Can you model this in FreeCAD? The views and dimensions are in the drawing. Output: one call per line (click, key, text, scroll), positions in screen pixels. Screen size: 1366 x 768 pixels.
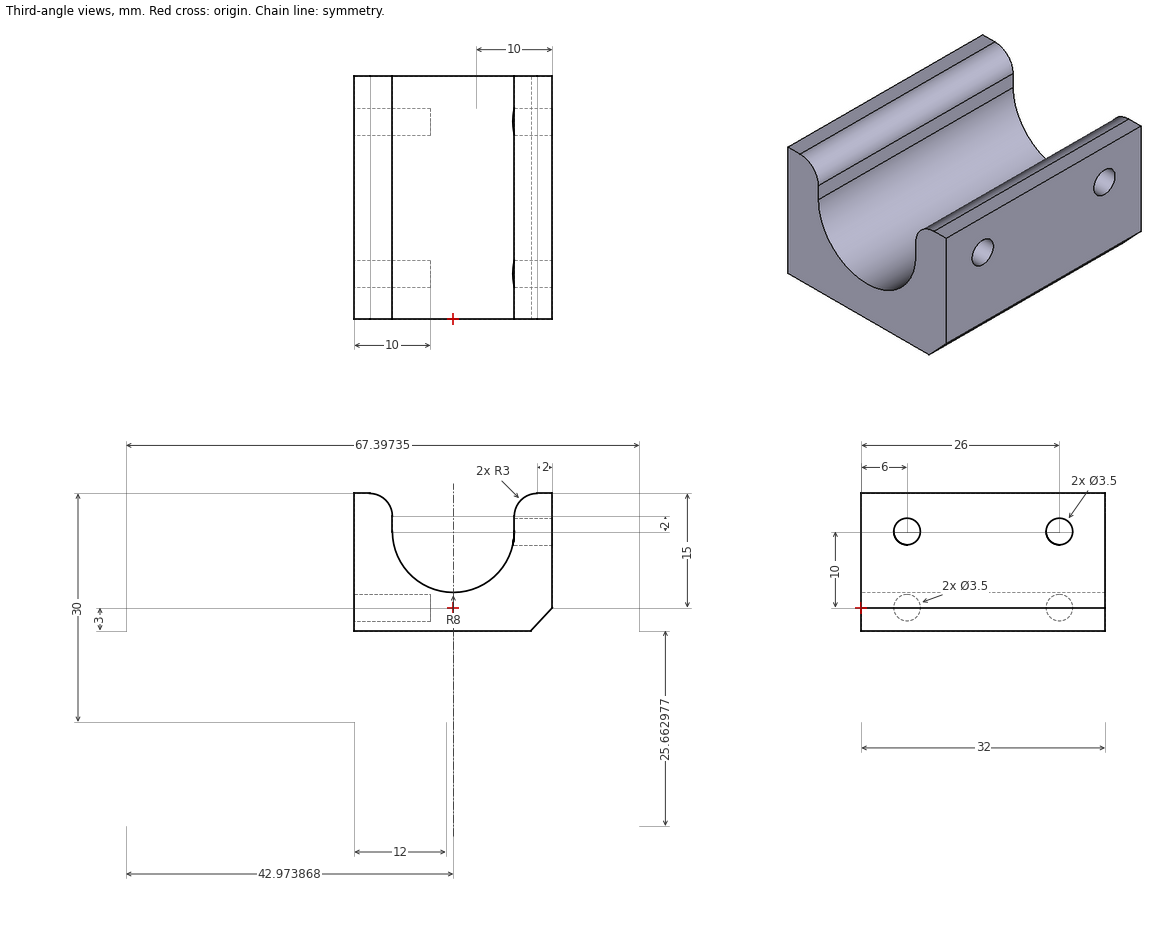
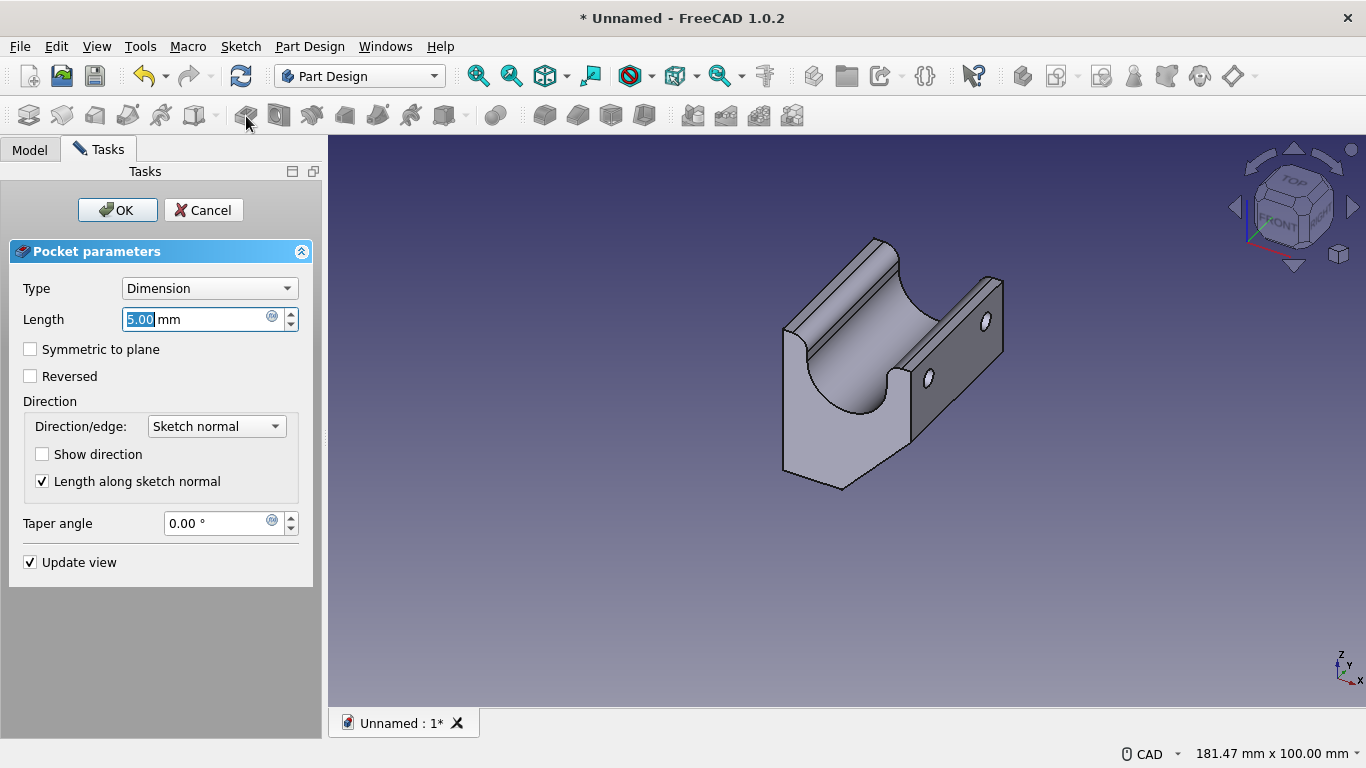
text(10)
key(Tab)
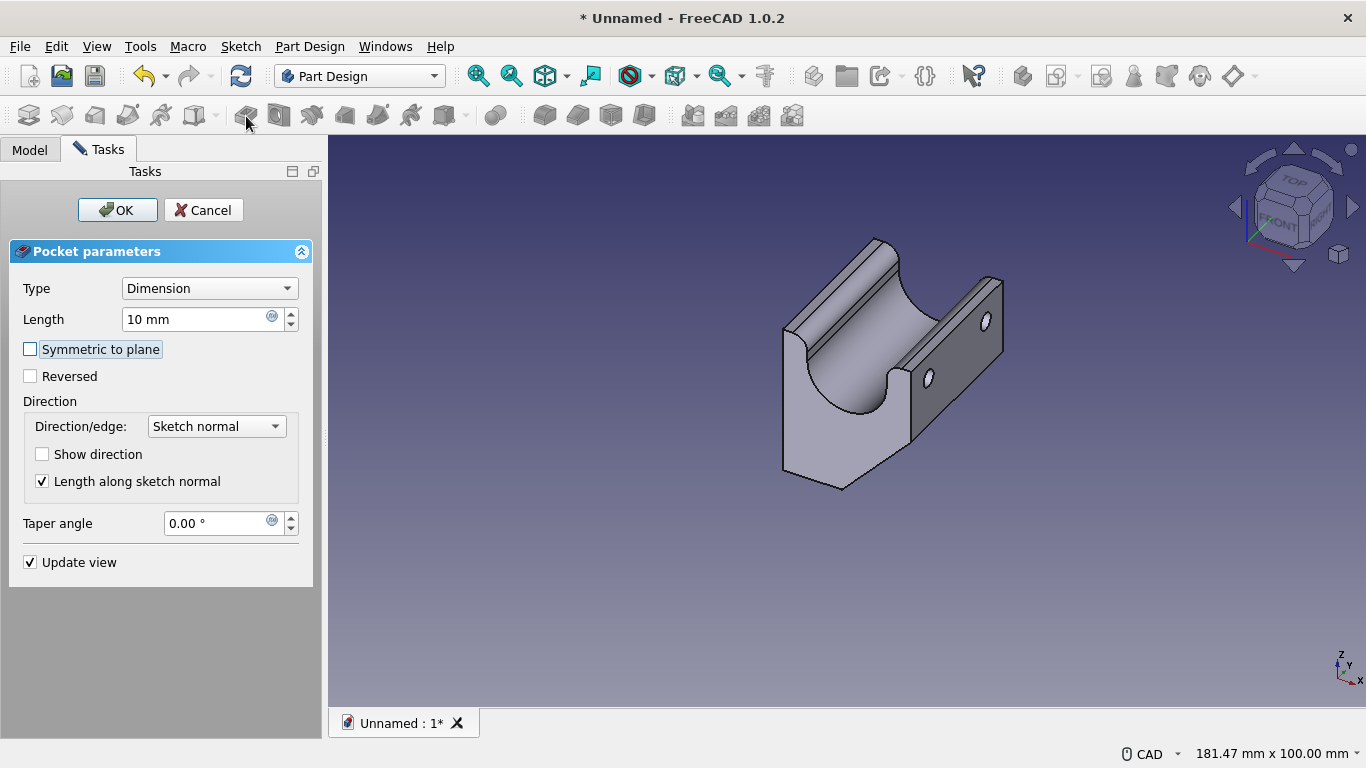
click(118, 210)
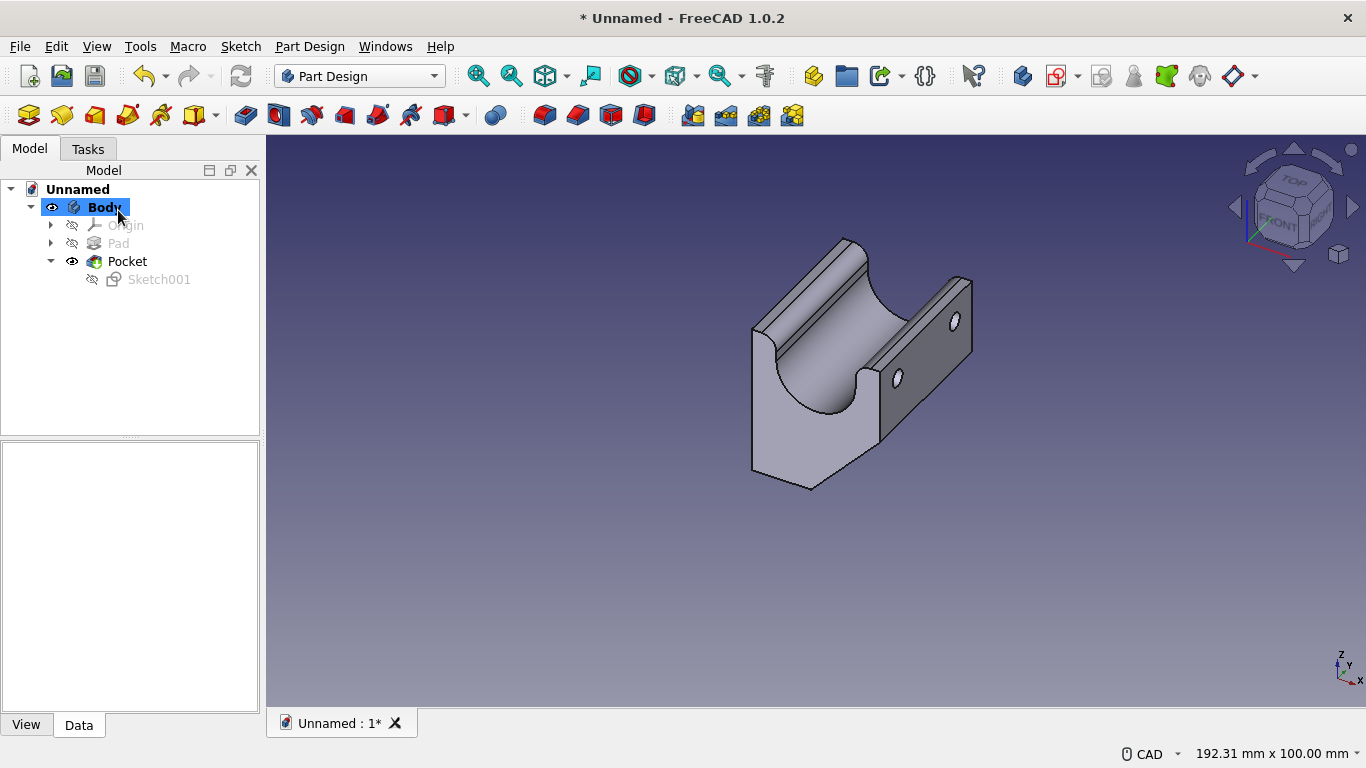
key(4)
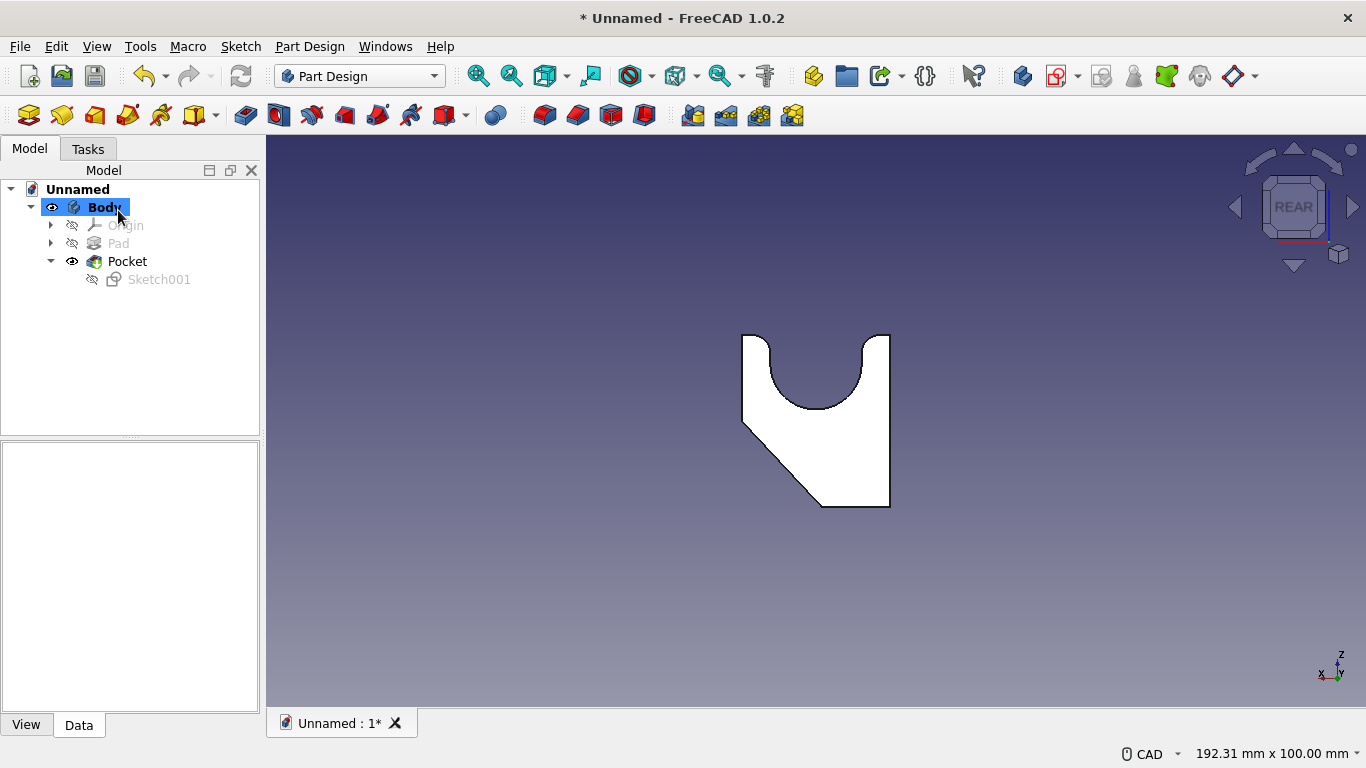
click(479, 76)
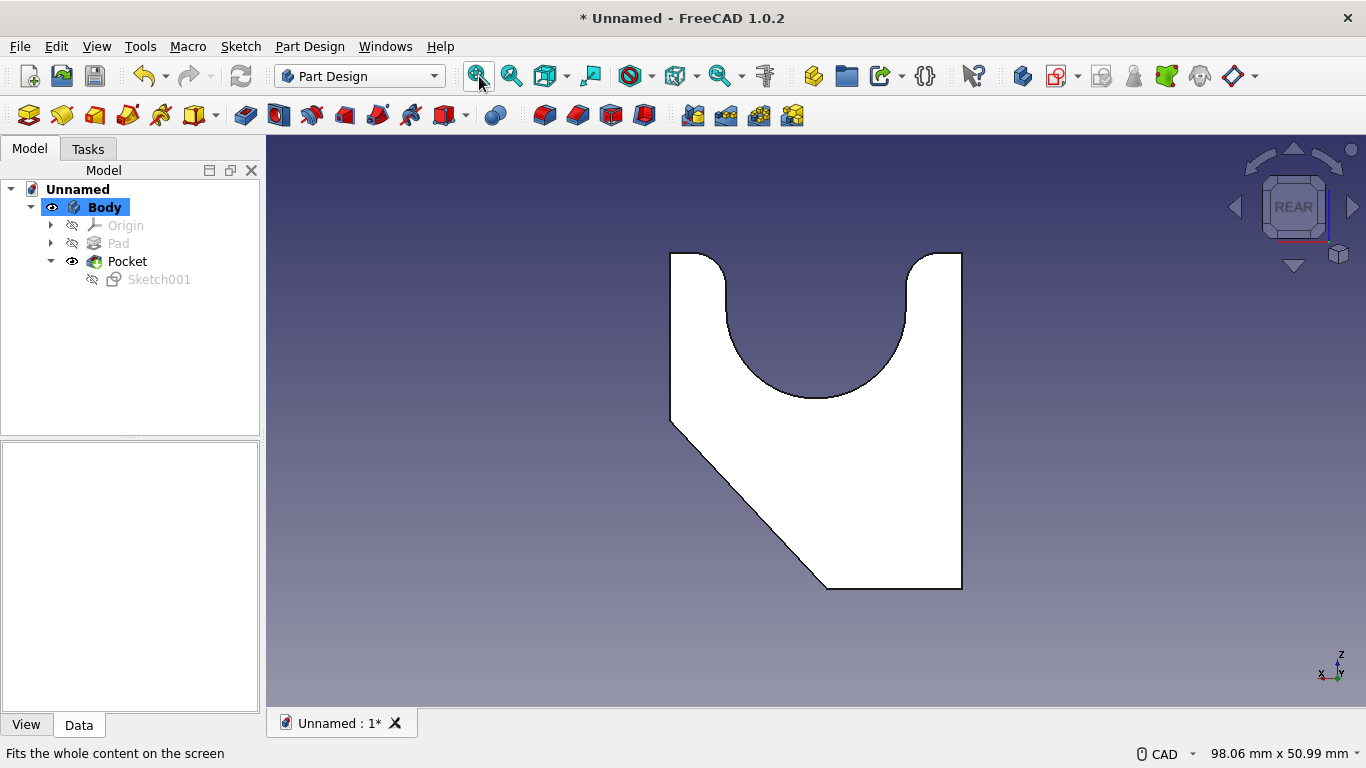
click(858, 468)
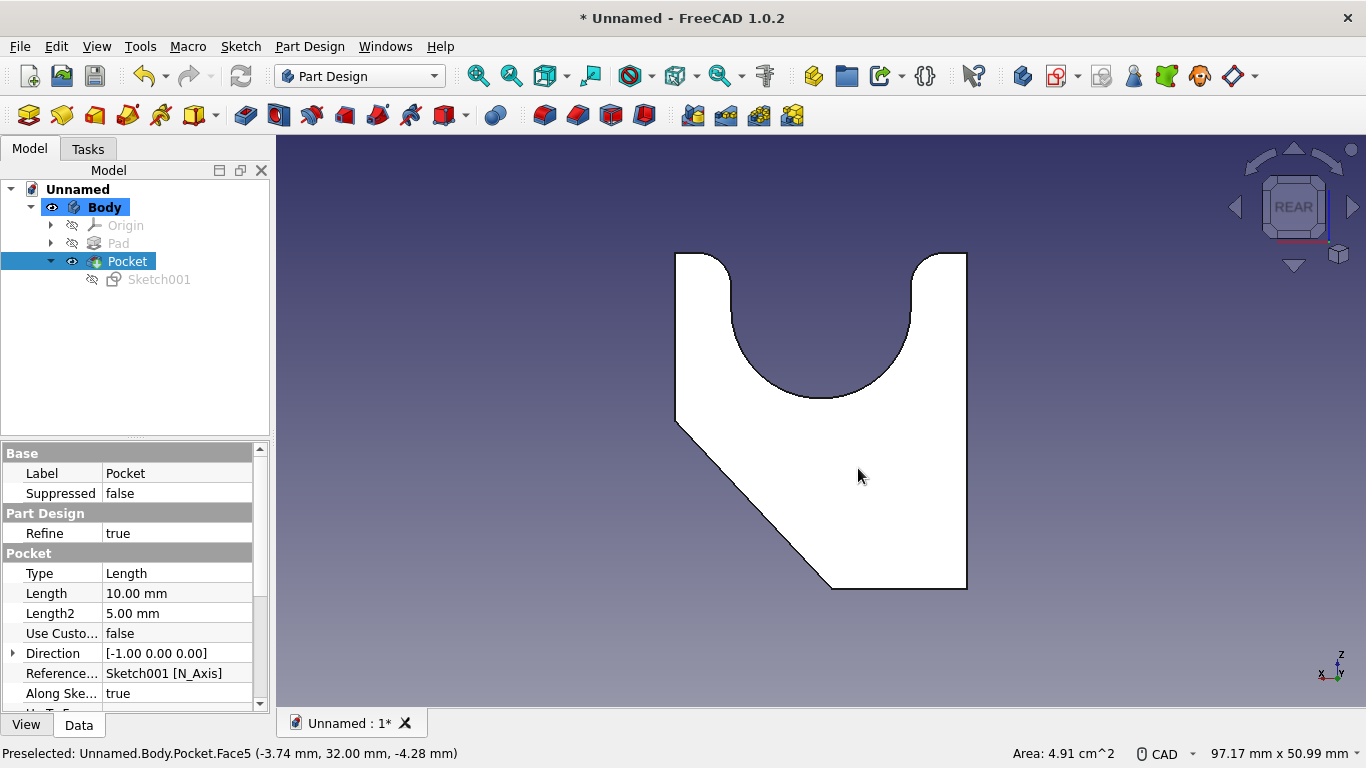
click(1056, 76)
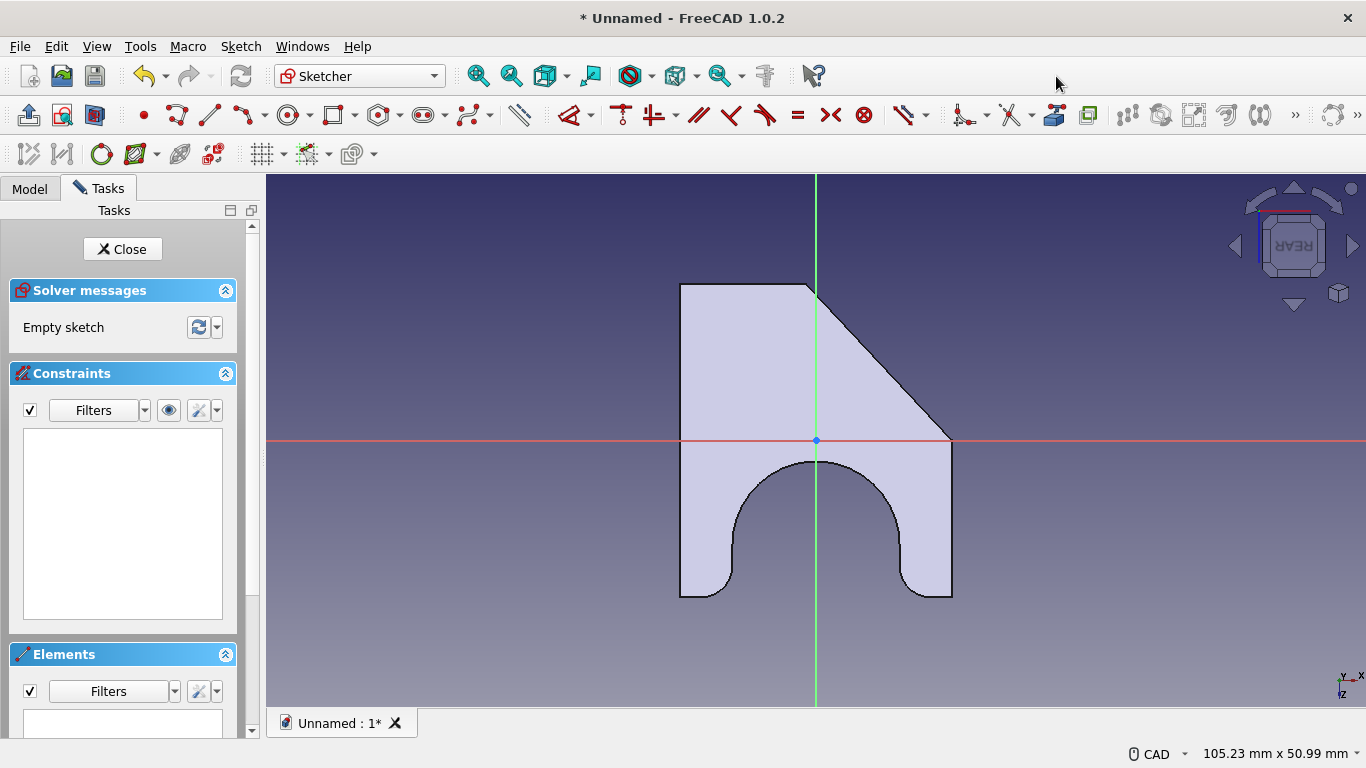
scroll(876, 679, down, 1)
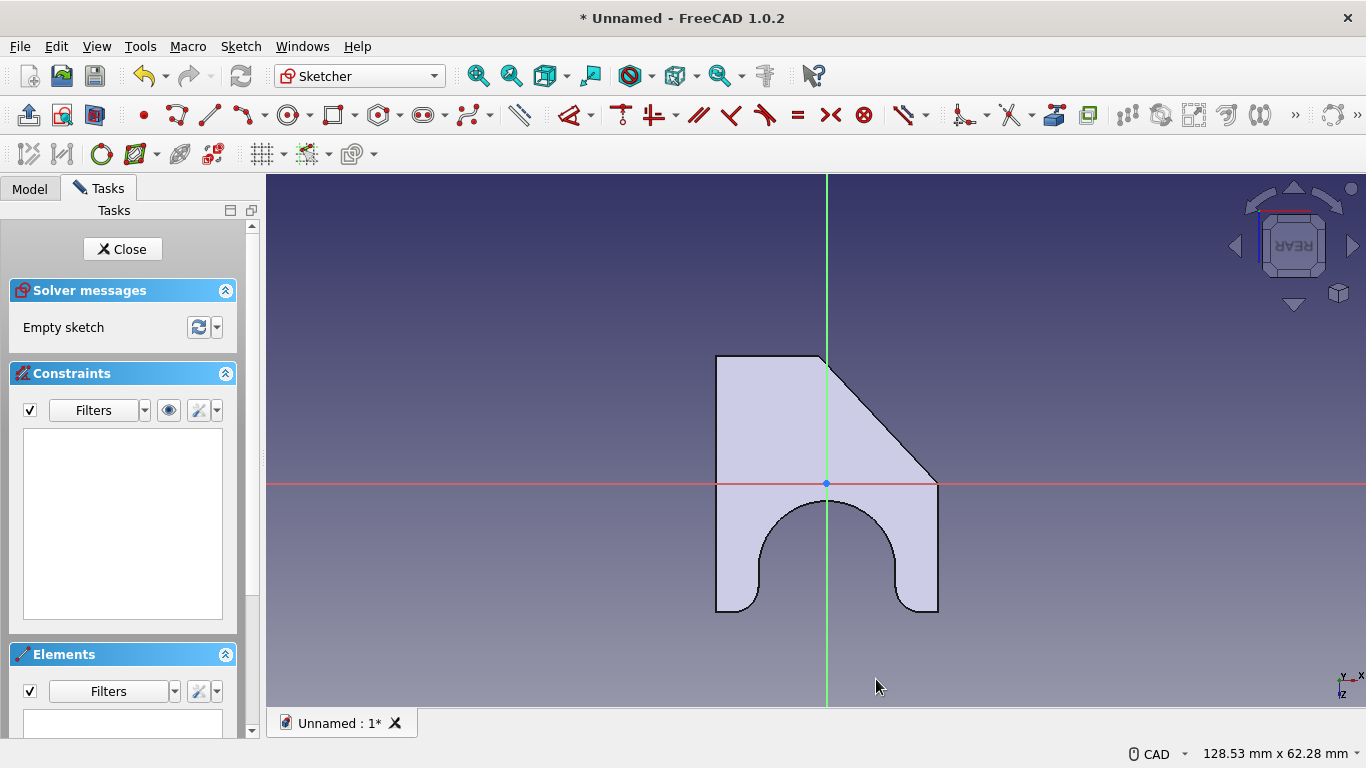
click(332, 116)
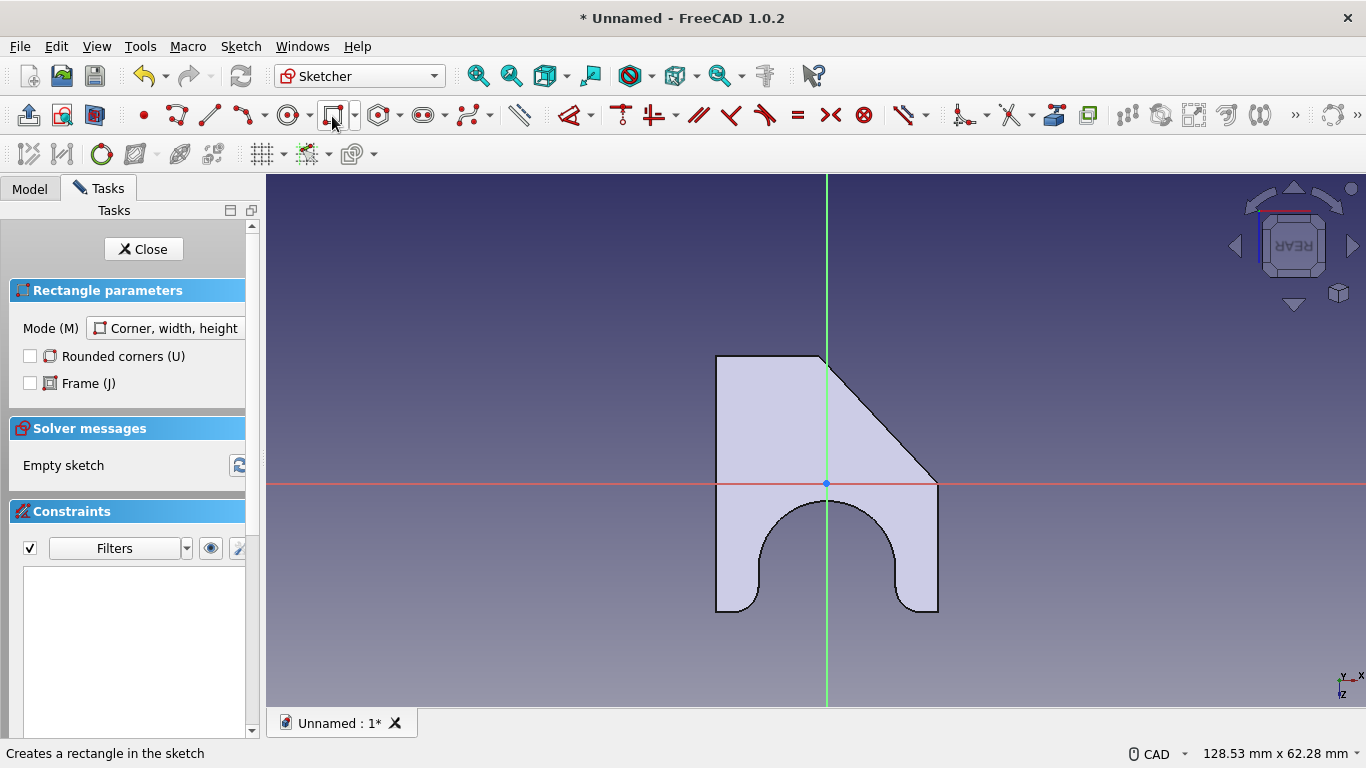
click(459, 239)
move(1036, 458)